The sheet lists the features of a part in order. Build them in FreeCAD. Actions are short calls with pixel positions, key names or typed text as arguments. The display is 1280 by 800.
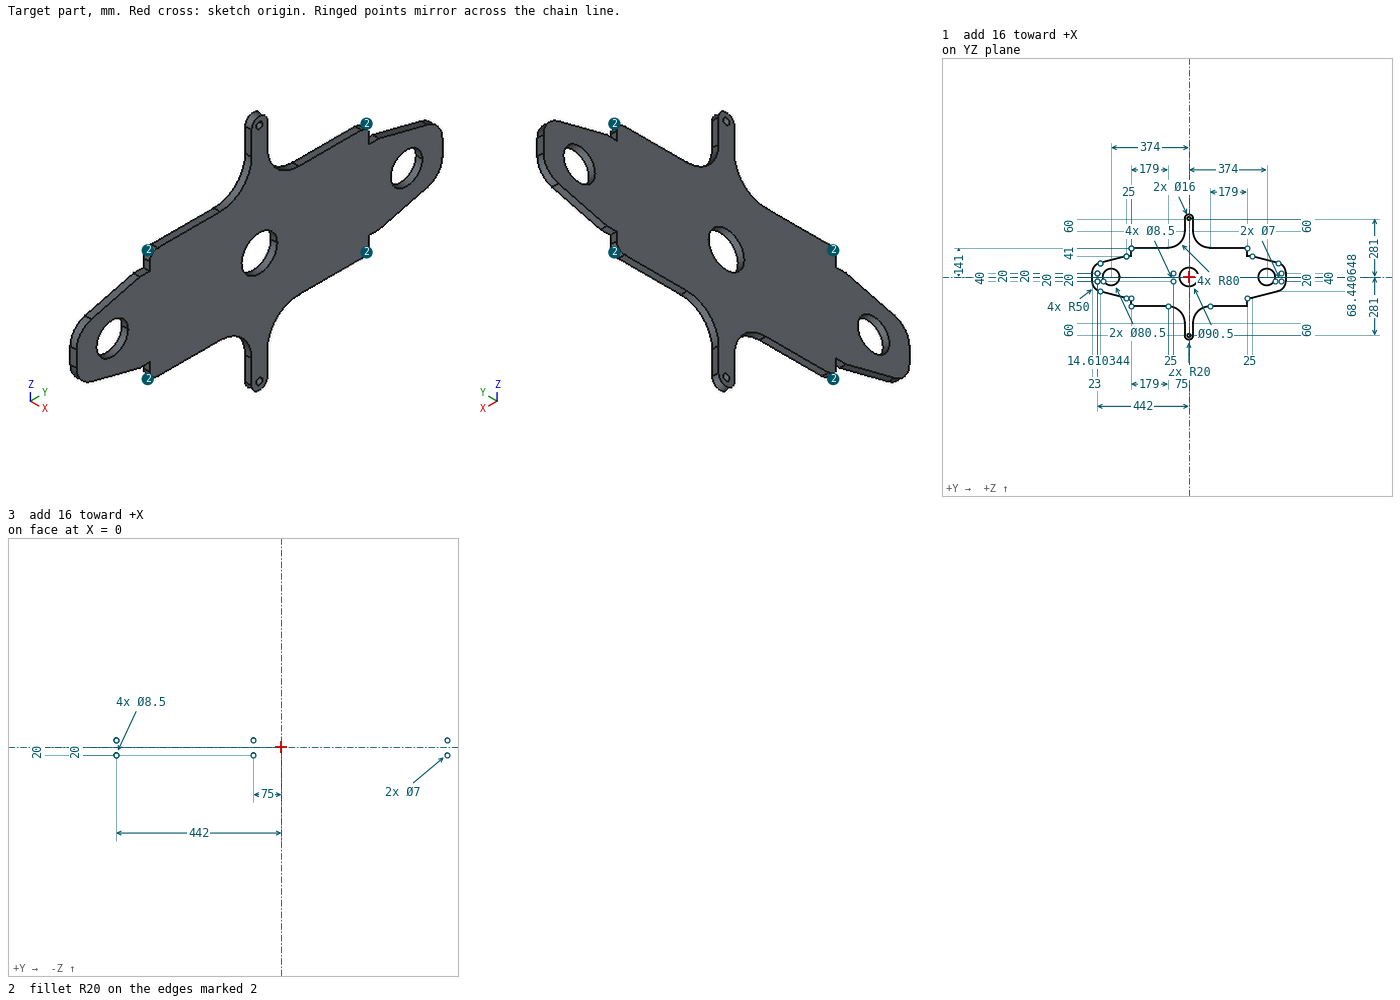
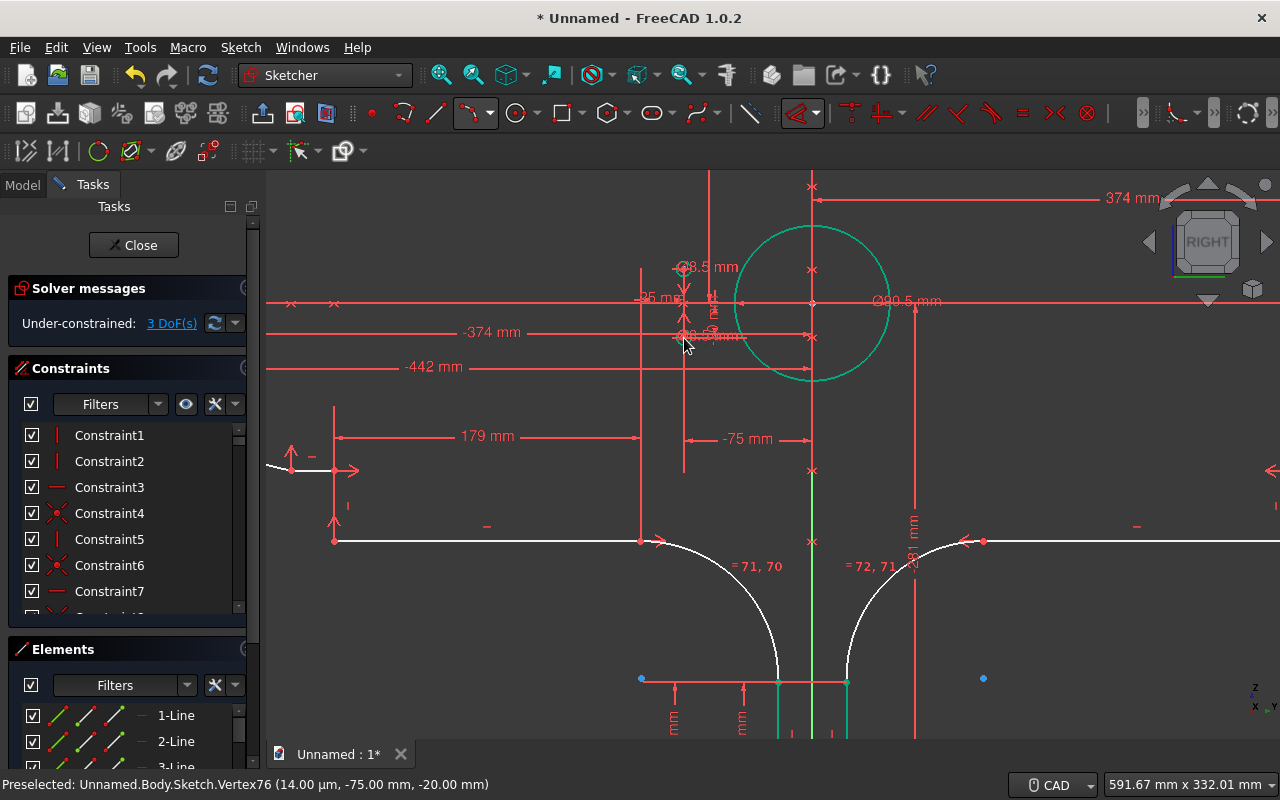
scroll(642, 542, down, 5)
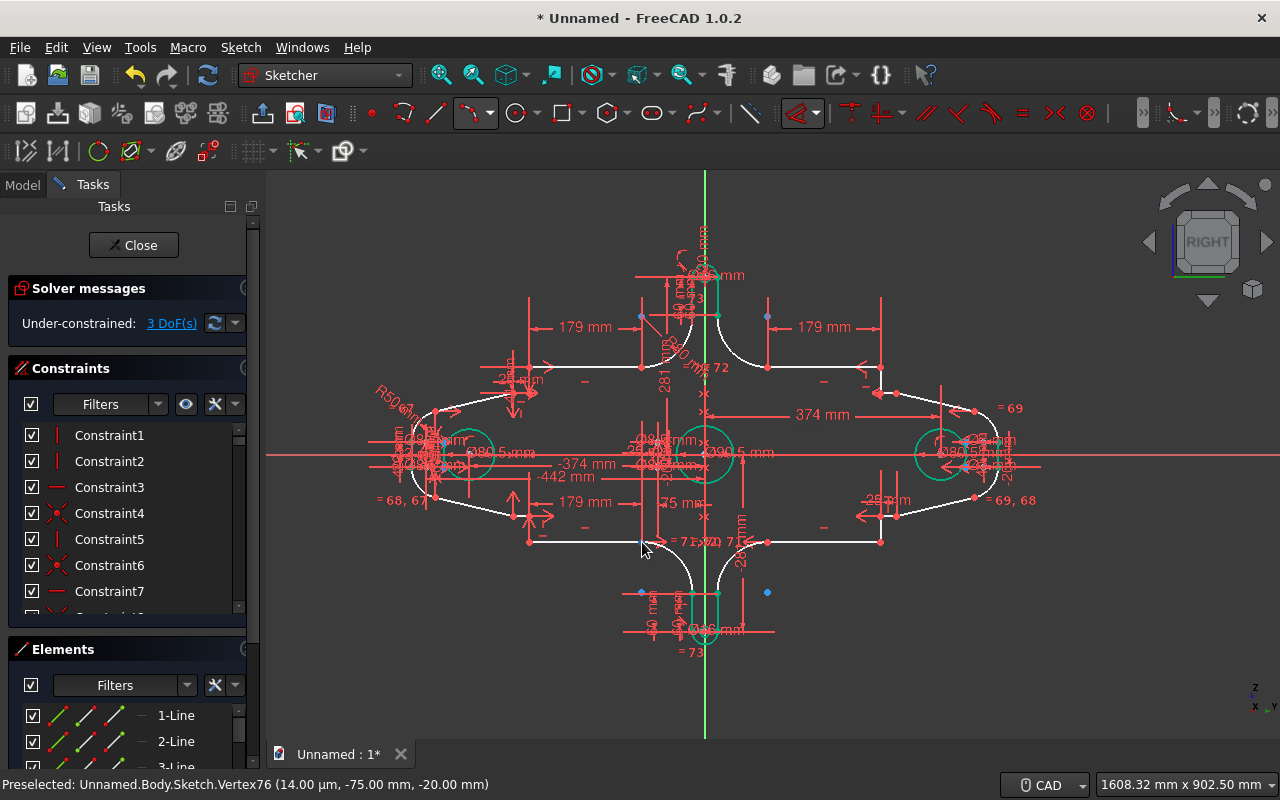
click(642, 367)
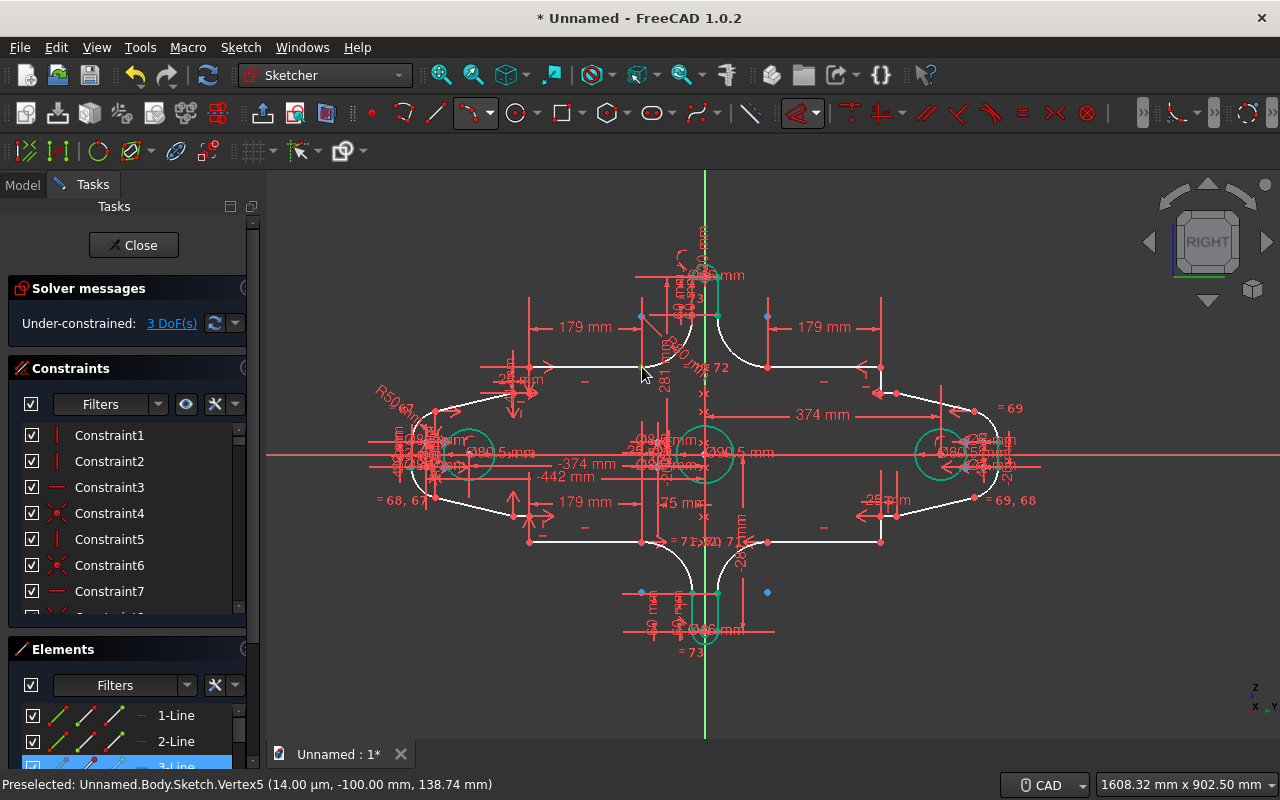
click(818, 114)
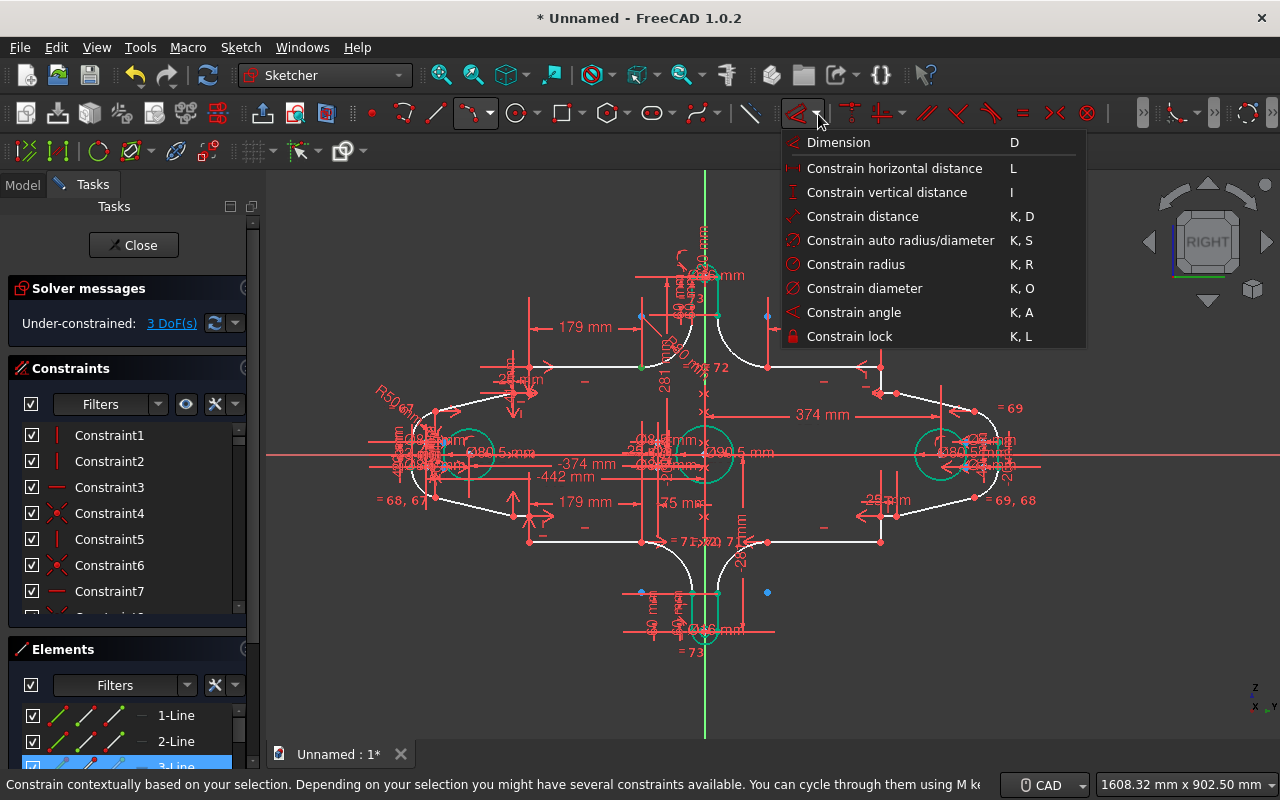
click(934, 192)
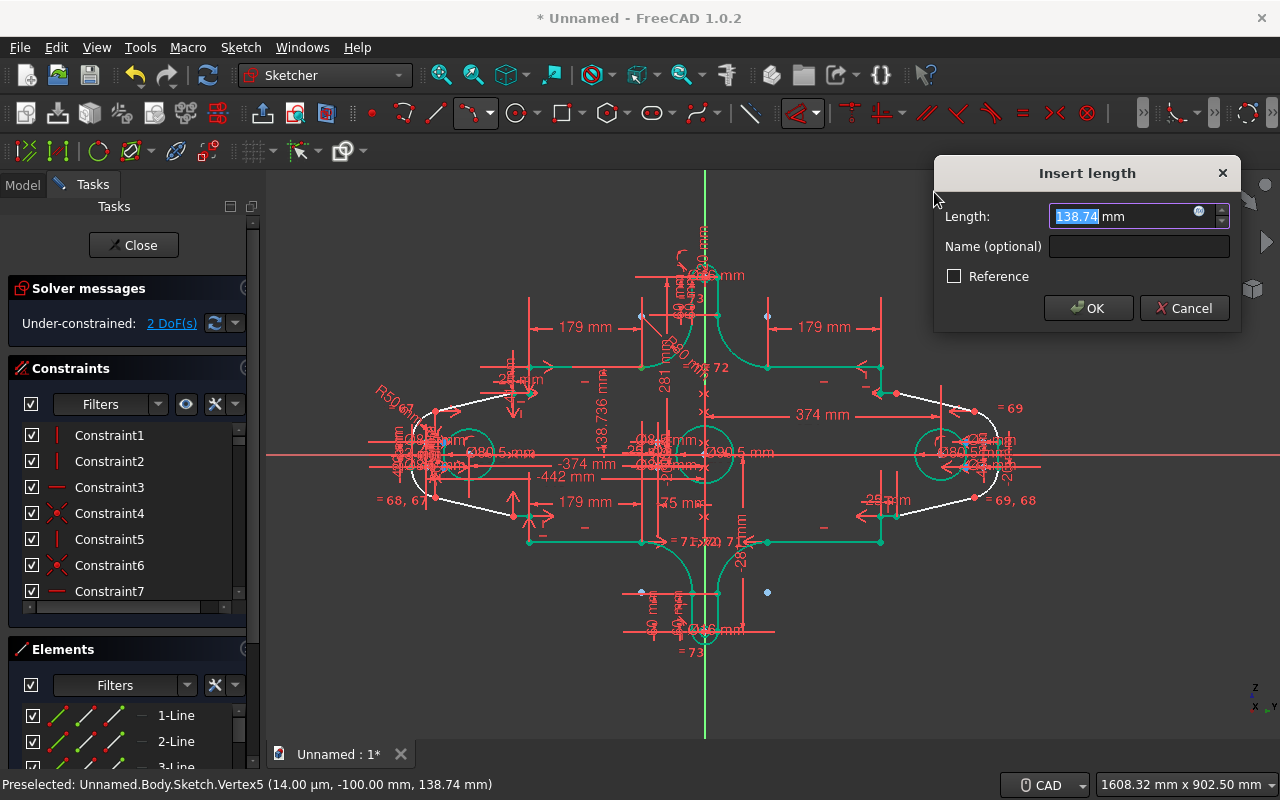
text(141)
key(Return)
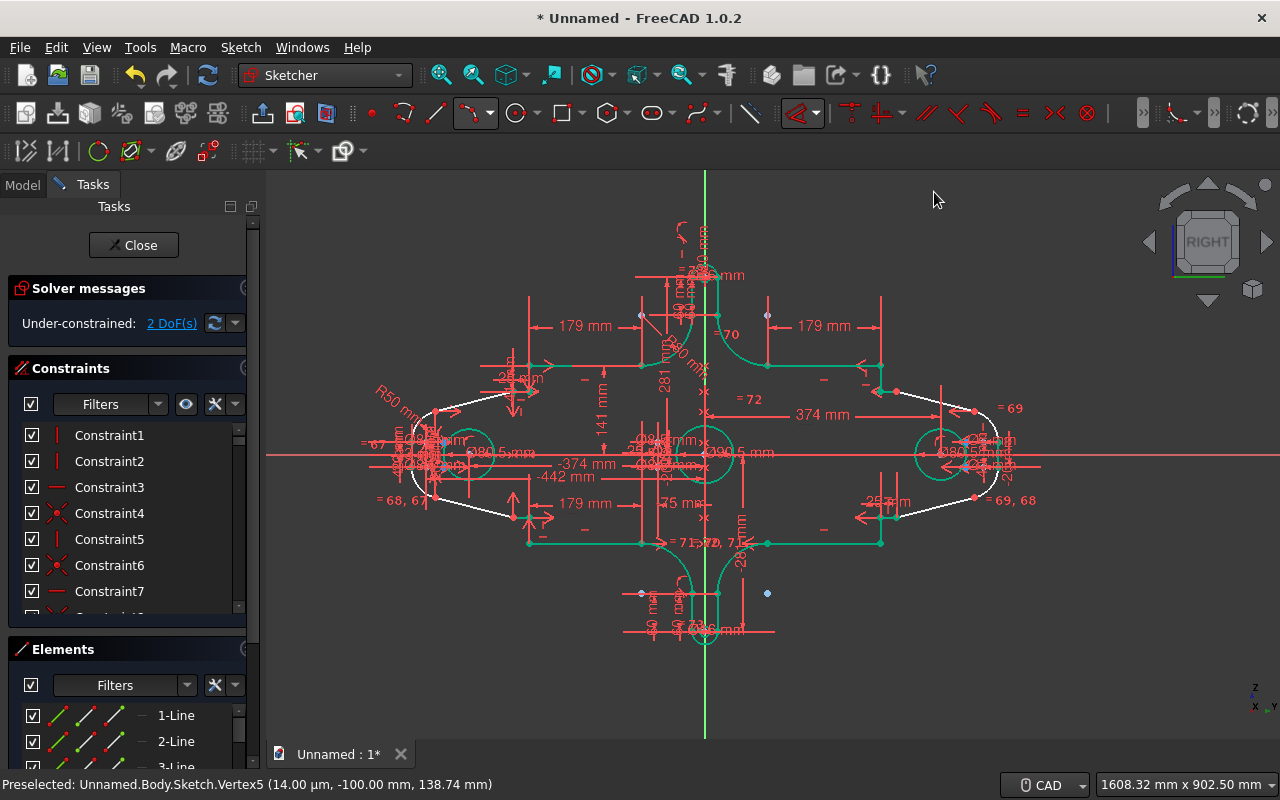
click(974, 498)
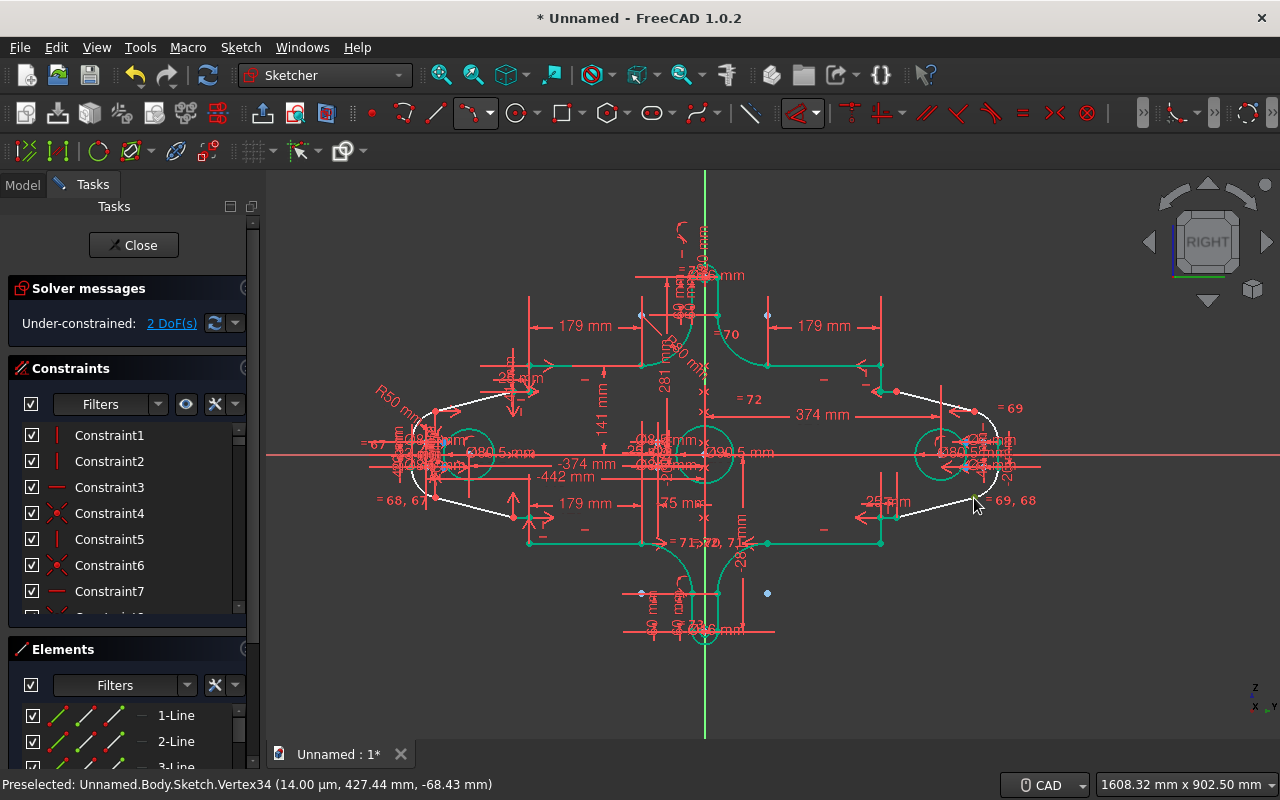
click(818, 114)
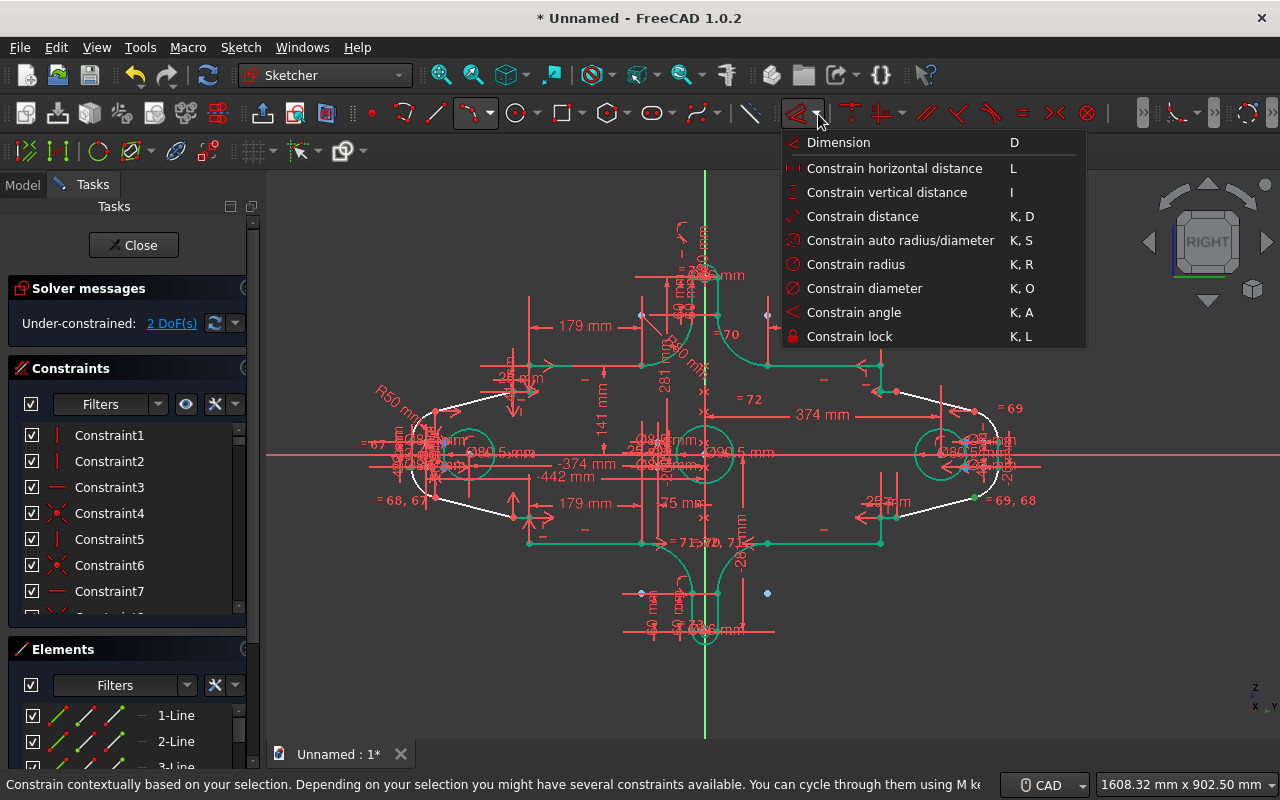
click(934, 192)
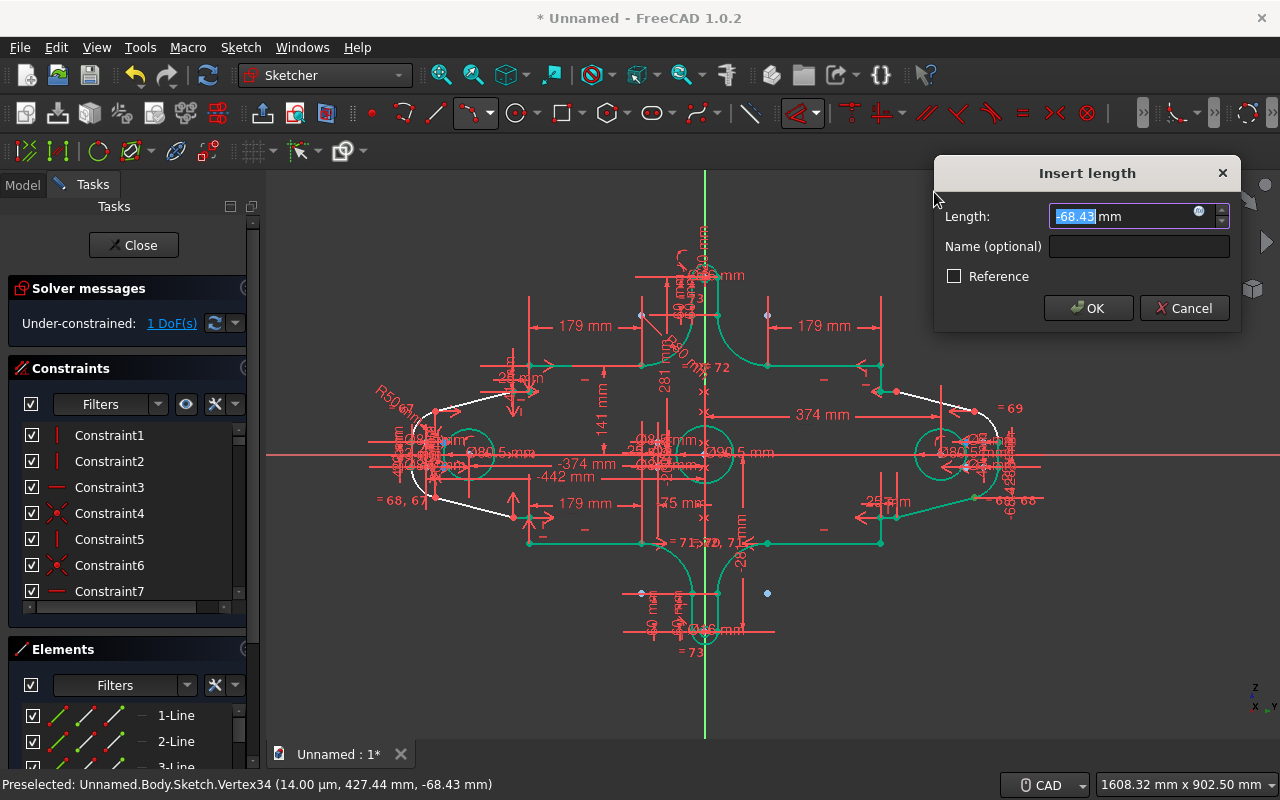
text(-68.440648)
key(Return)